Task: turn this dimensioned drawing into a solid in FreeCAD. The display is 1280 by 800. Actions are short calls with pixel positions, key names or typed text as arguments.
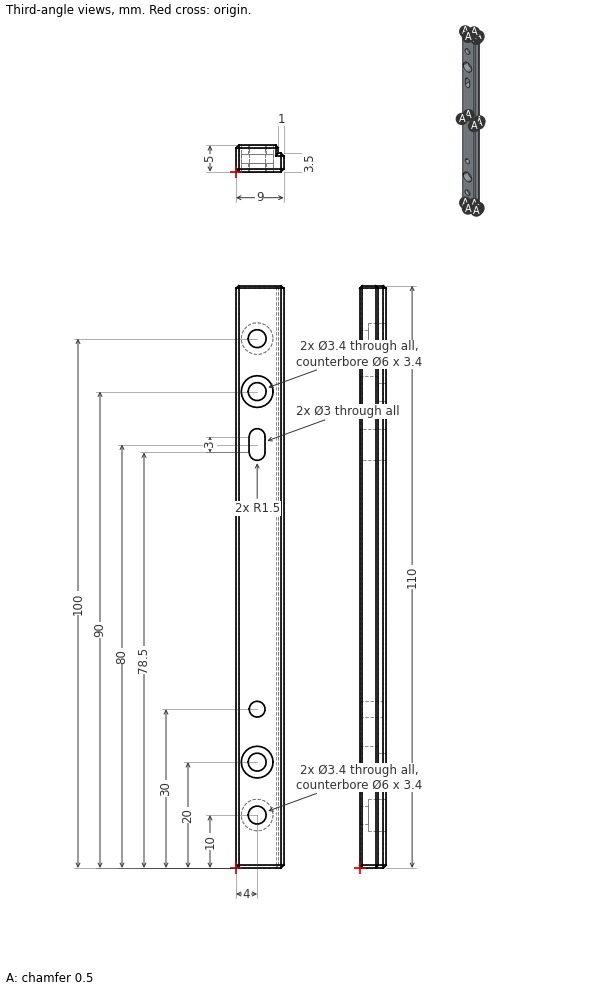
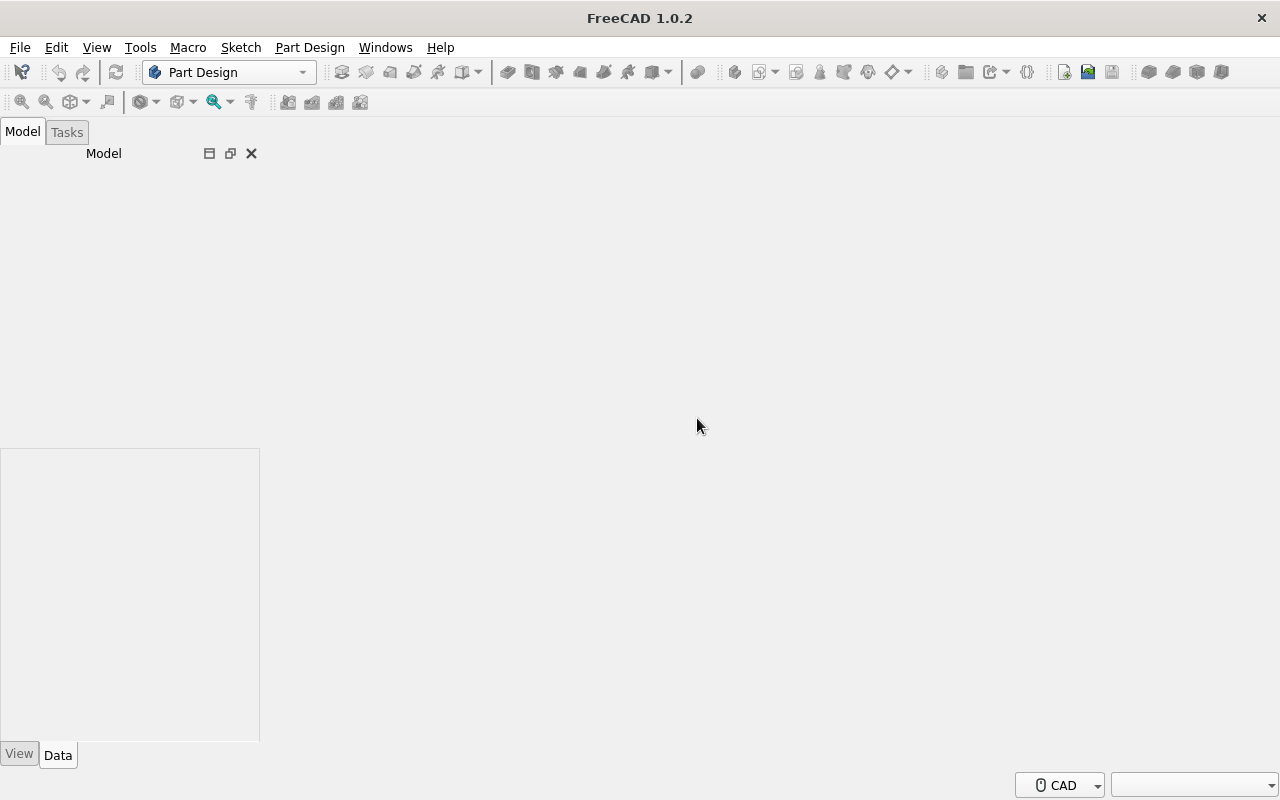
click(1064, 72)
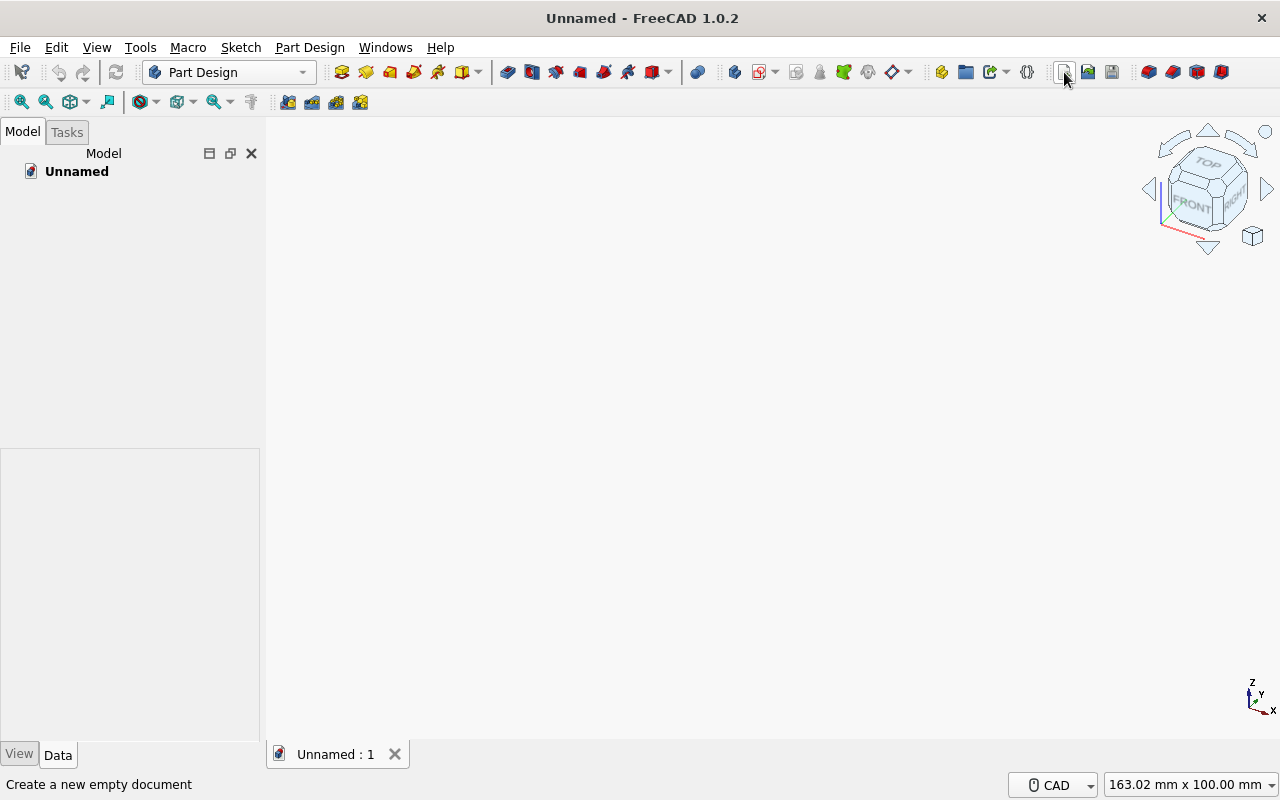
click(760, 72)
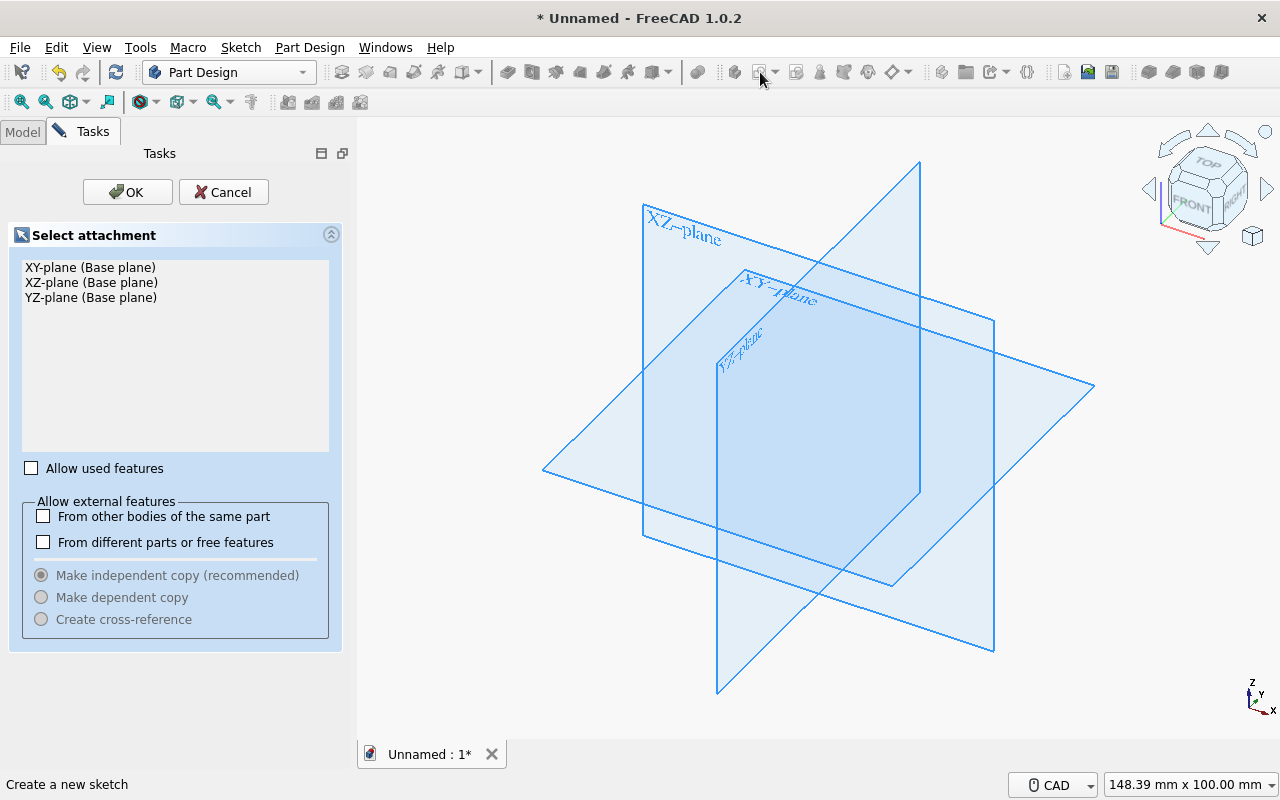
click(82, 268)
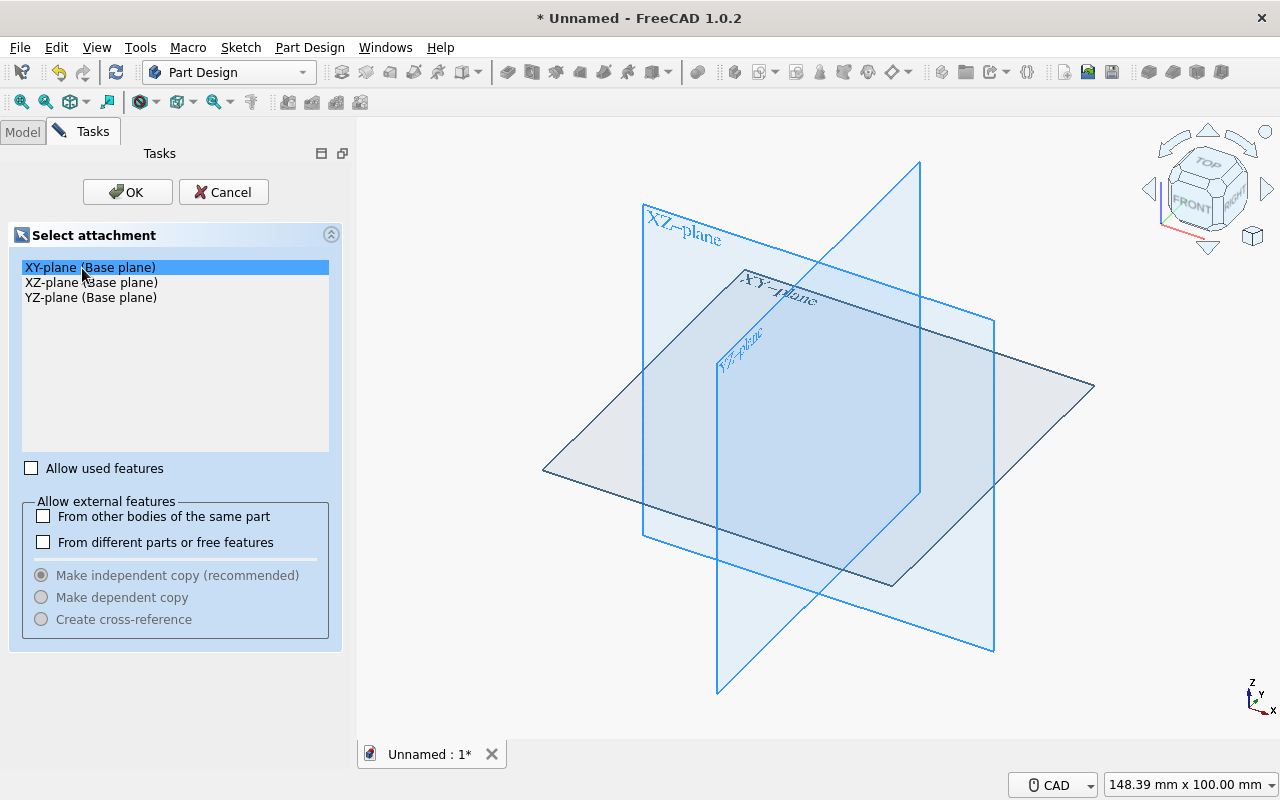
click(128, 192)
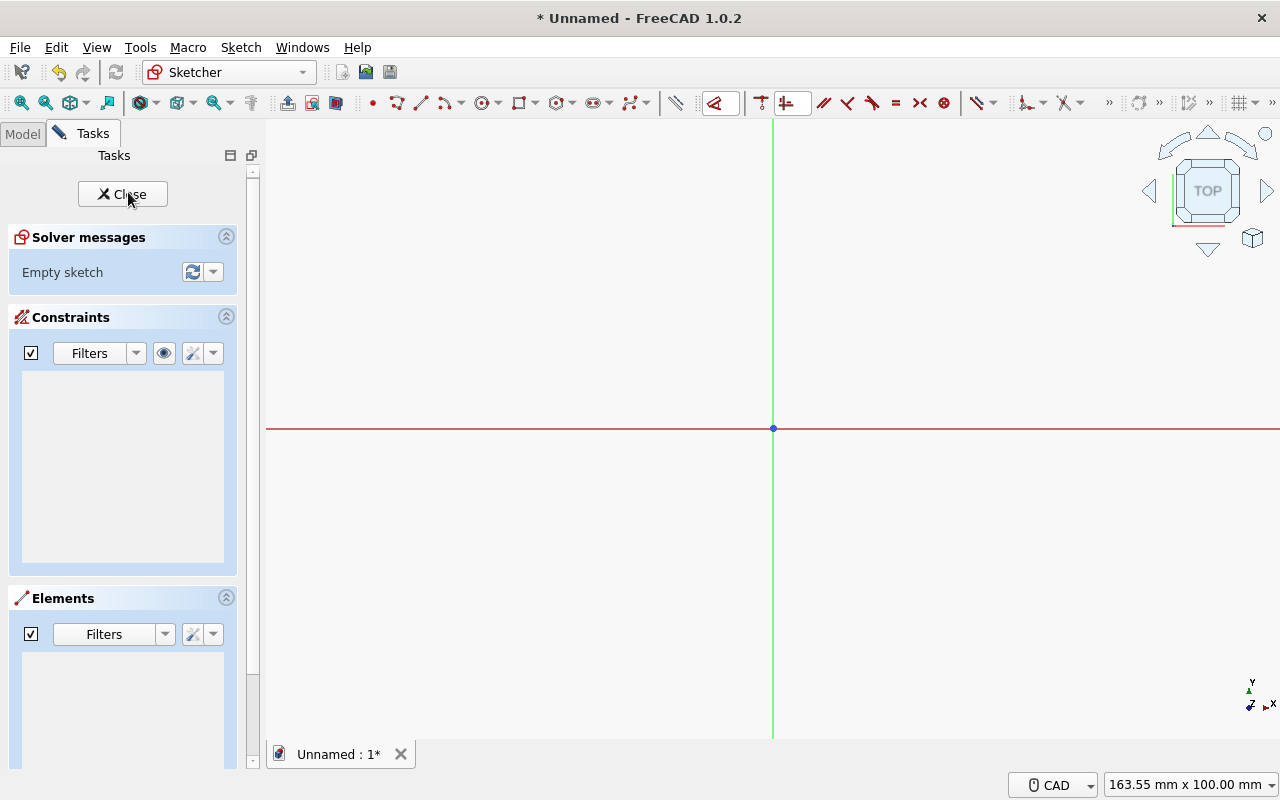
scroll(811, 412, up, 12)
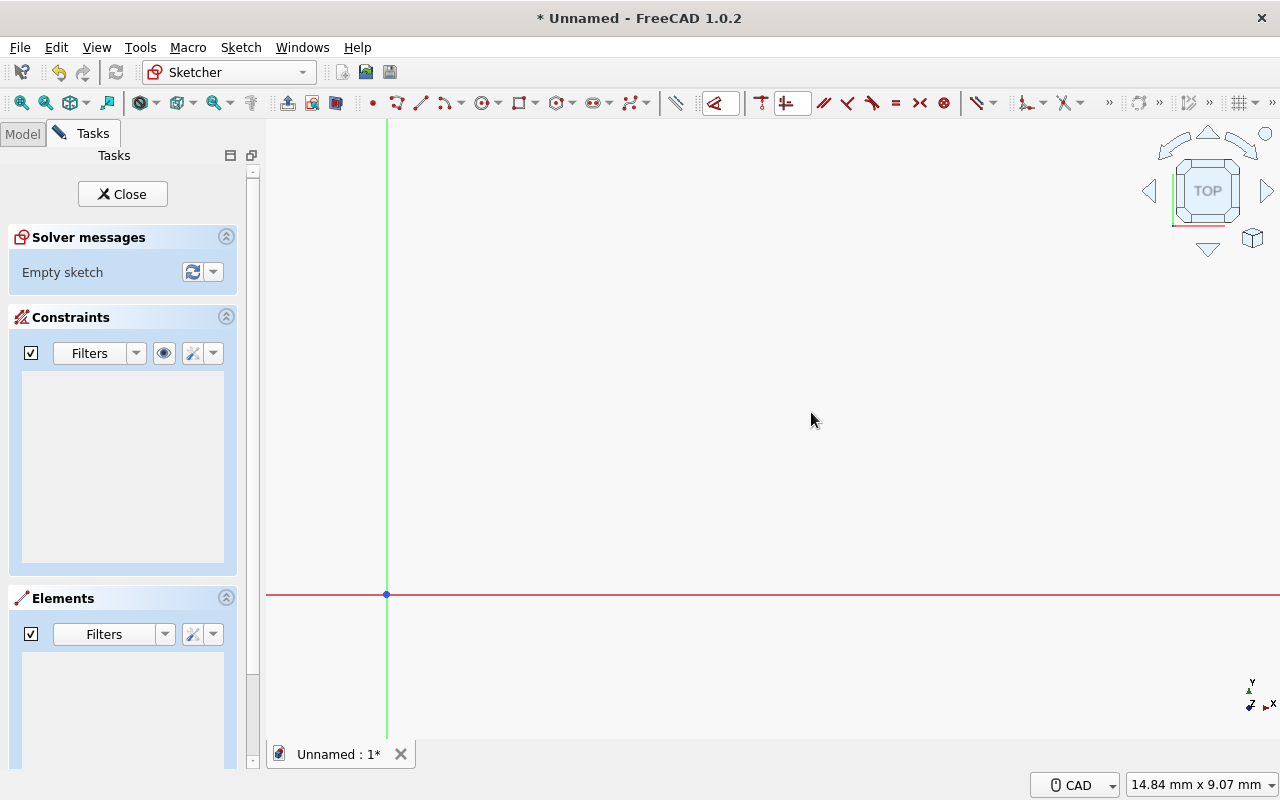
click(398, 104)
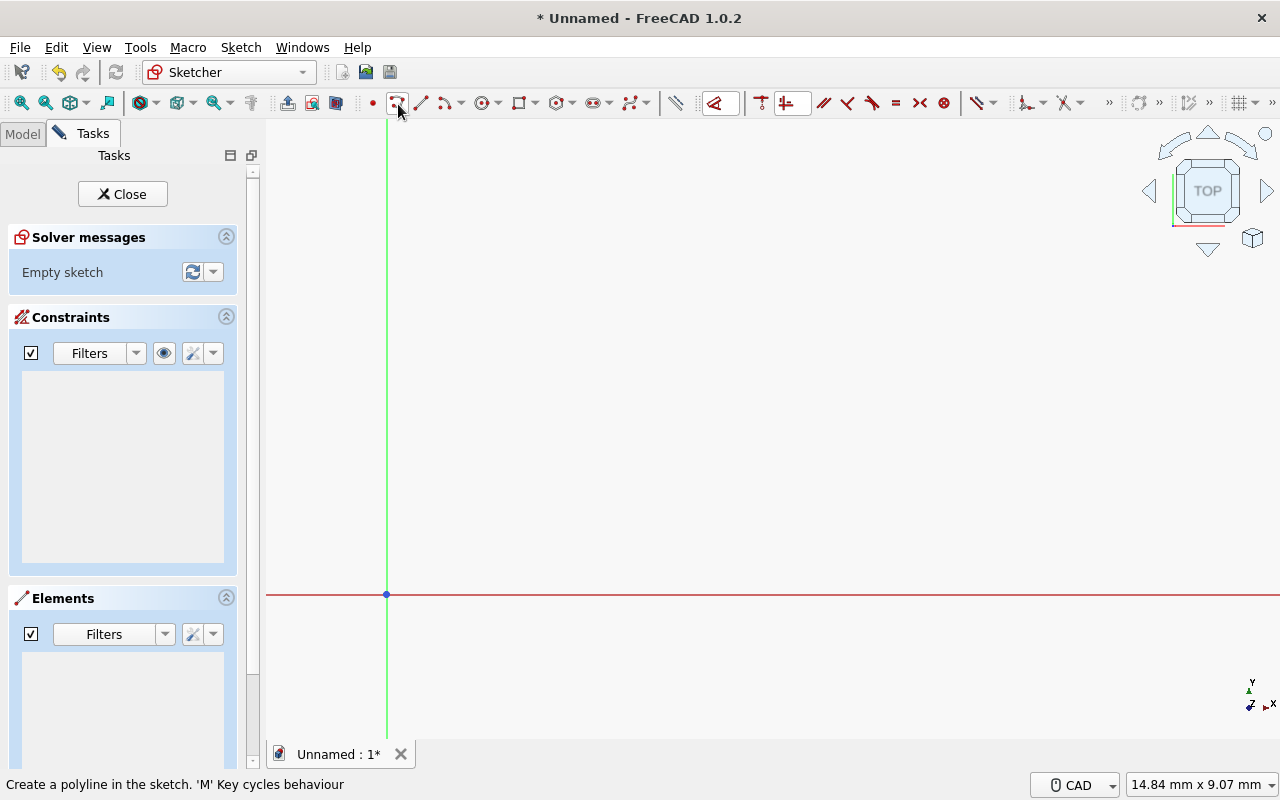
click(387, 595)
click(1002, 586)
click(1002, 355)
click(933, 355)
click(933, 253)
click(396, 253)
click(387, 595)
key(Escape)
key(Escape)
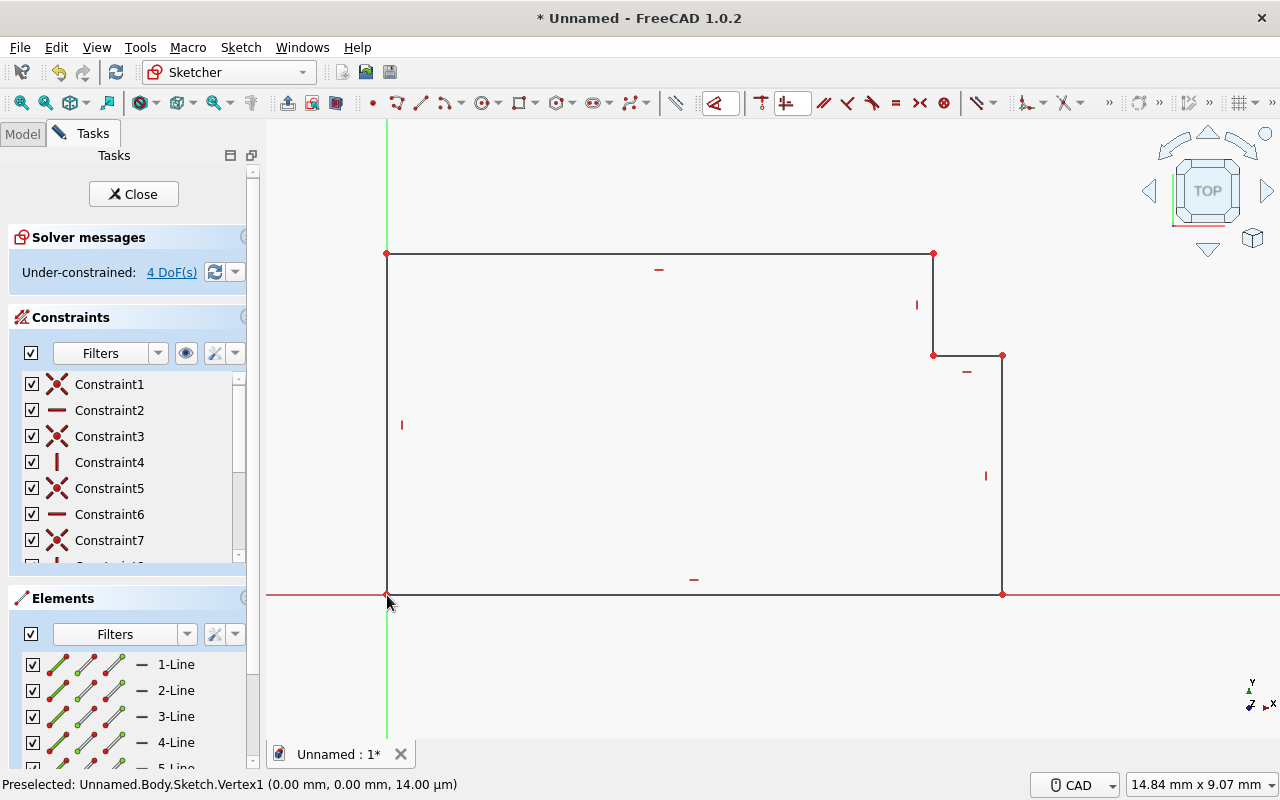
key(d)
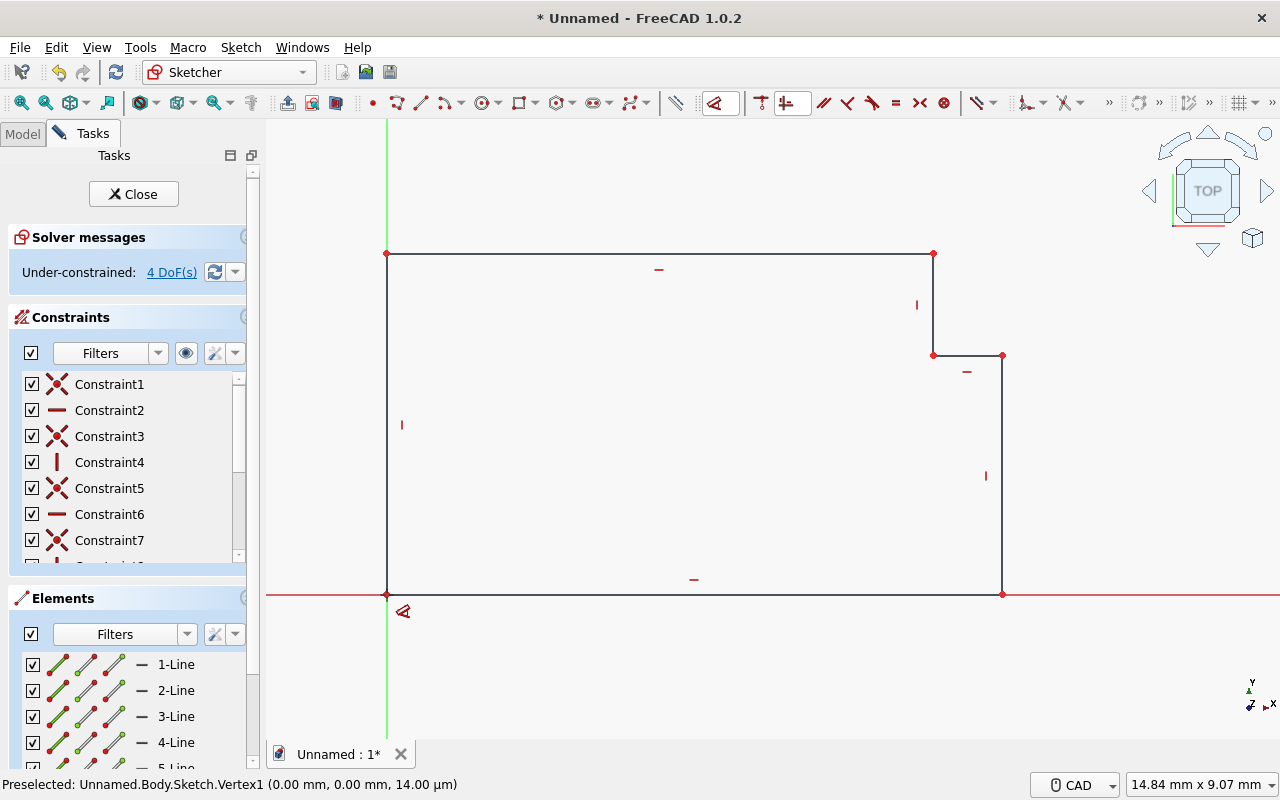
click(571, 595)
click(694, 629)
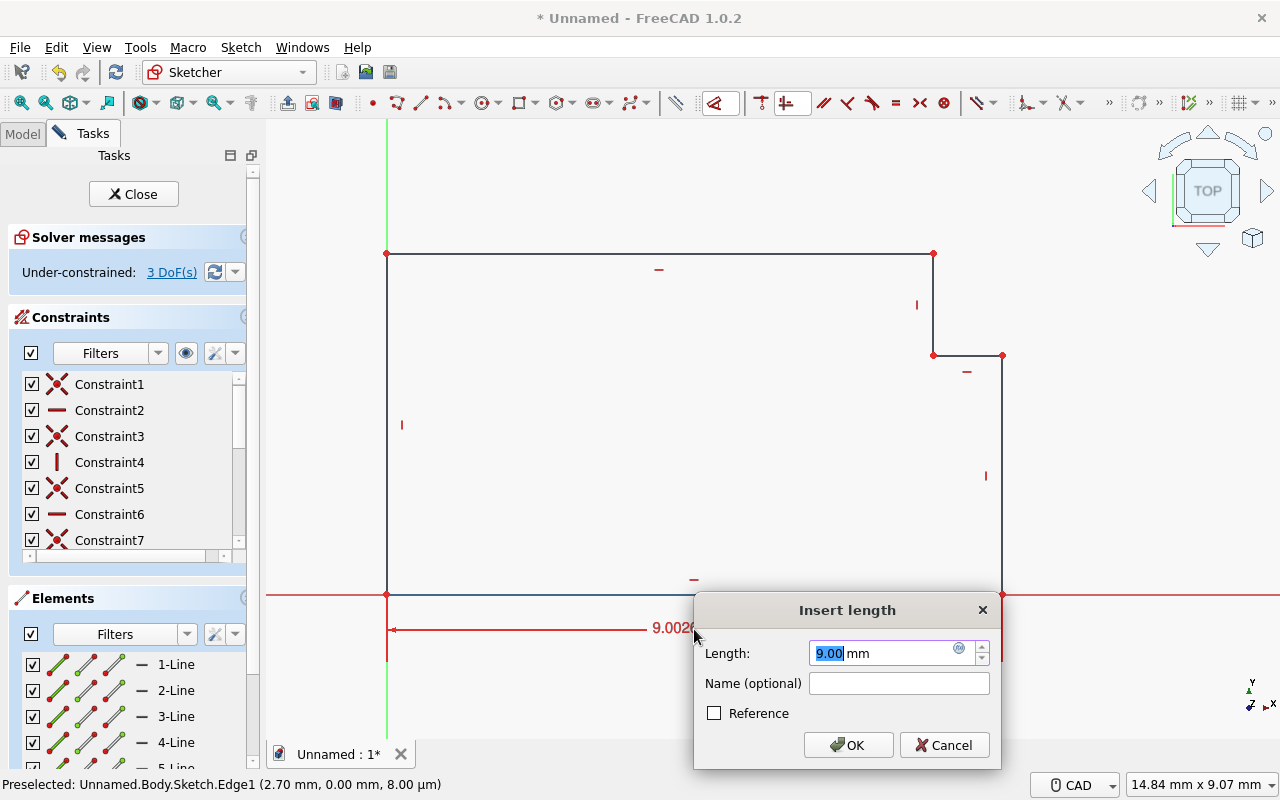
text(9)
key(Return)